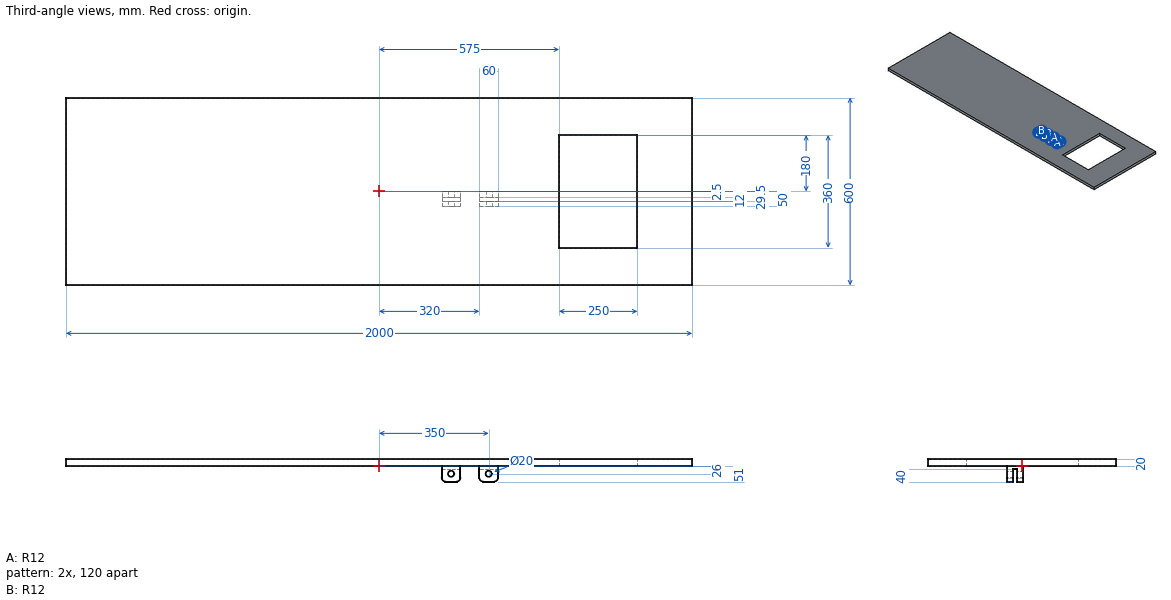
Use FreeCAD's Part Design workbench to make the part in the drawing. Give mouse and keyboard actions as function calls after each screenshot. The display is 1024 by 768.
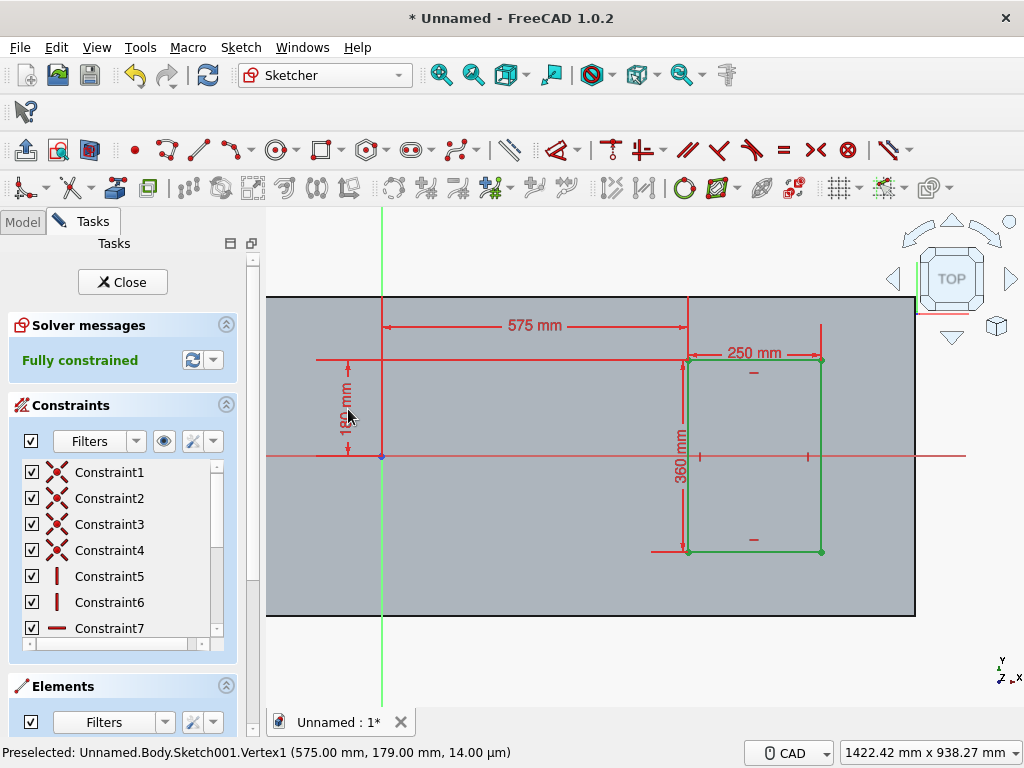
click(123, 282)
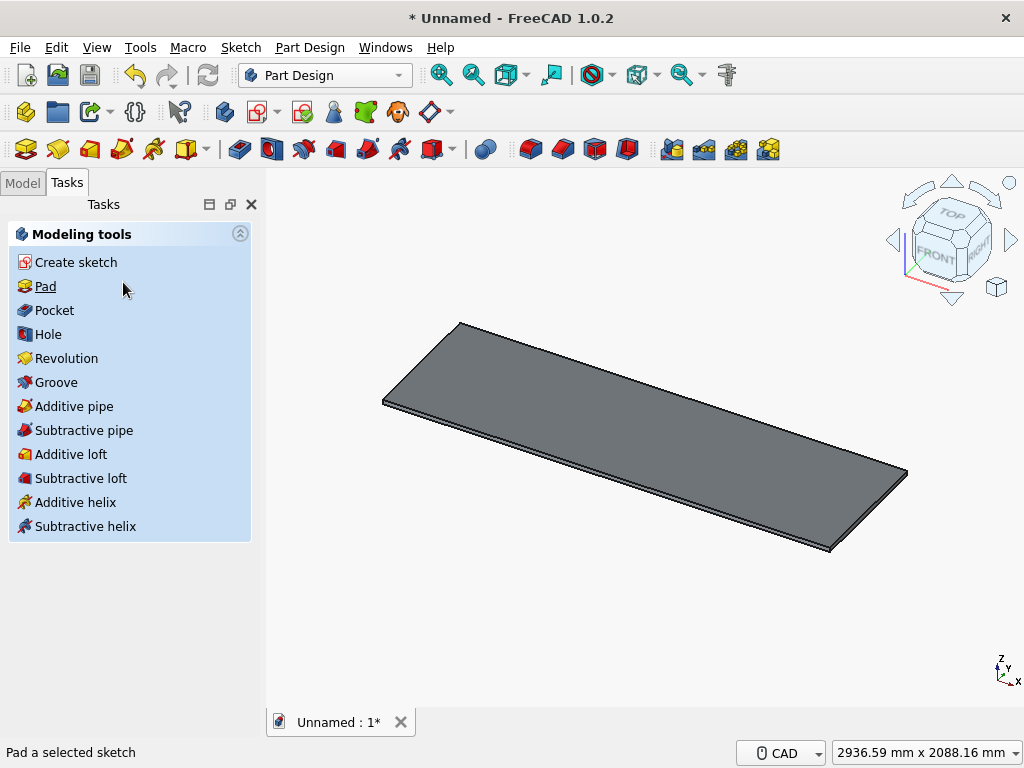
click(240, 150)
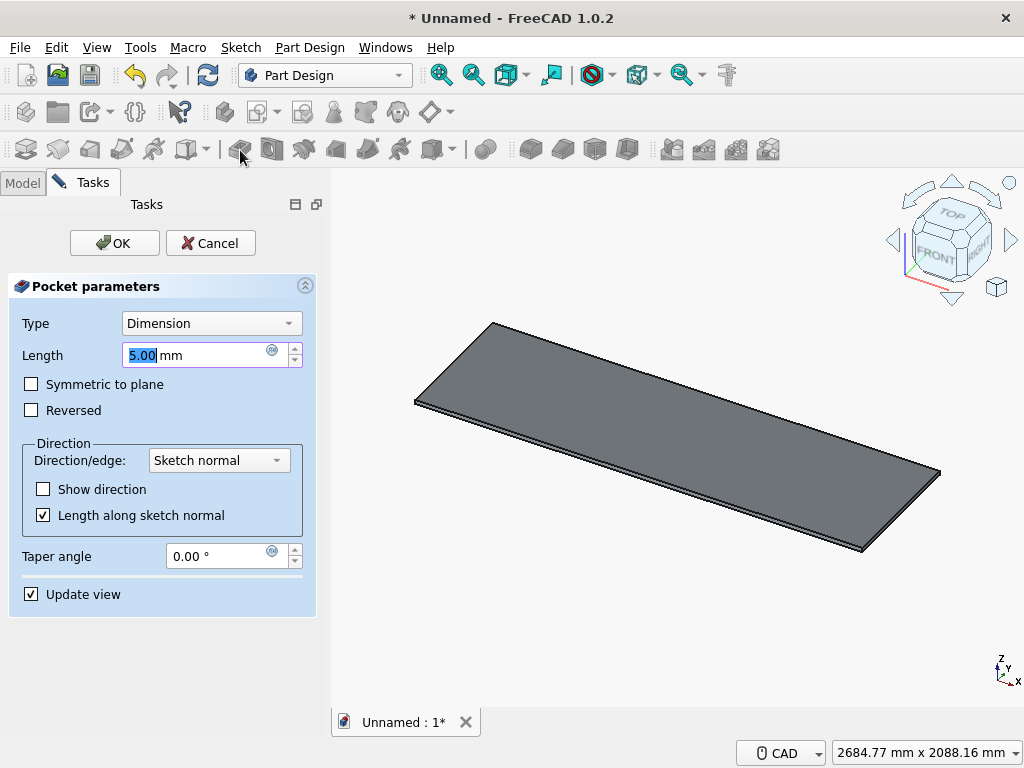
click(212, 324)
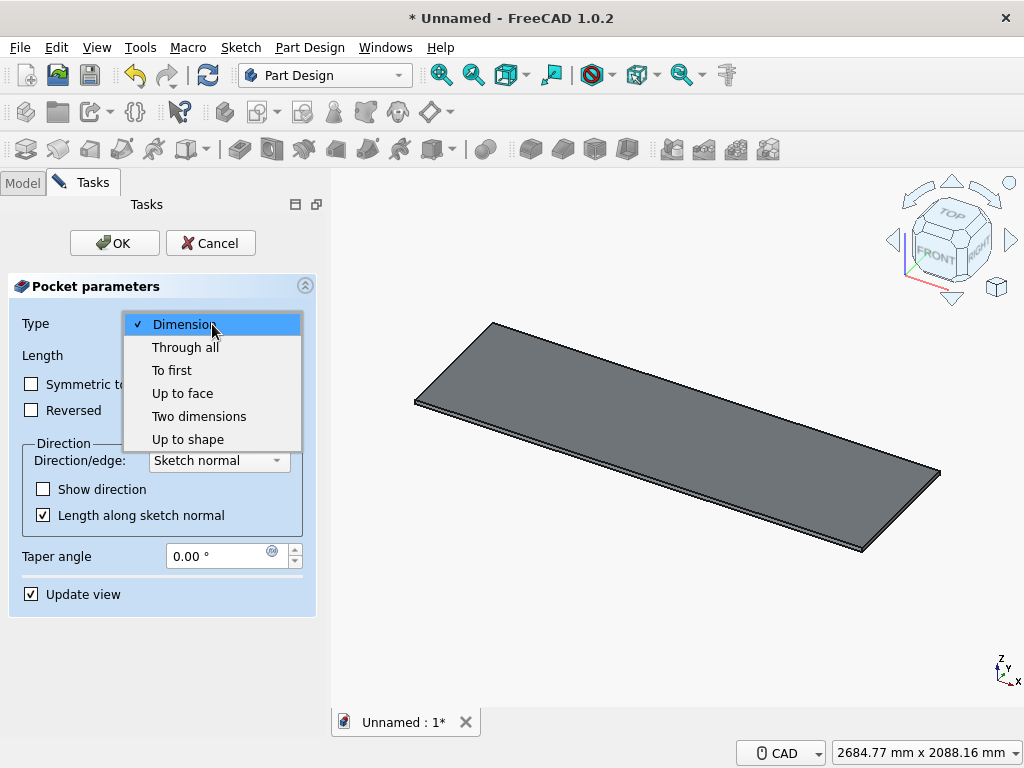
click(212, 348)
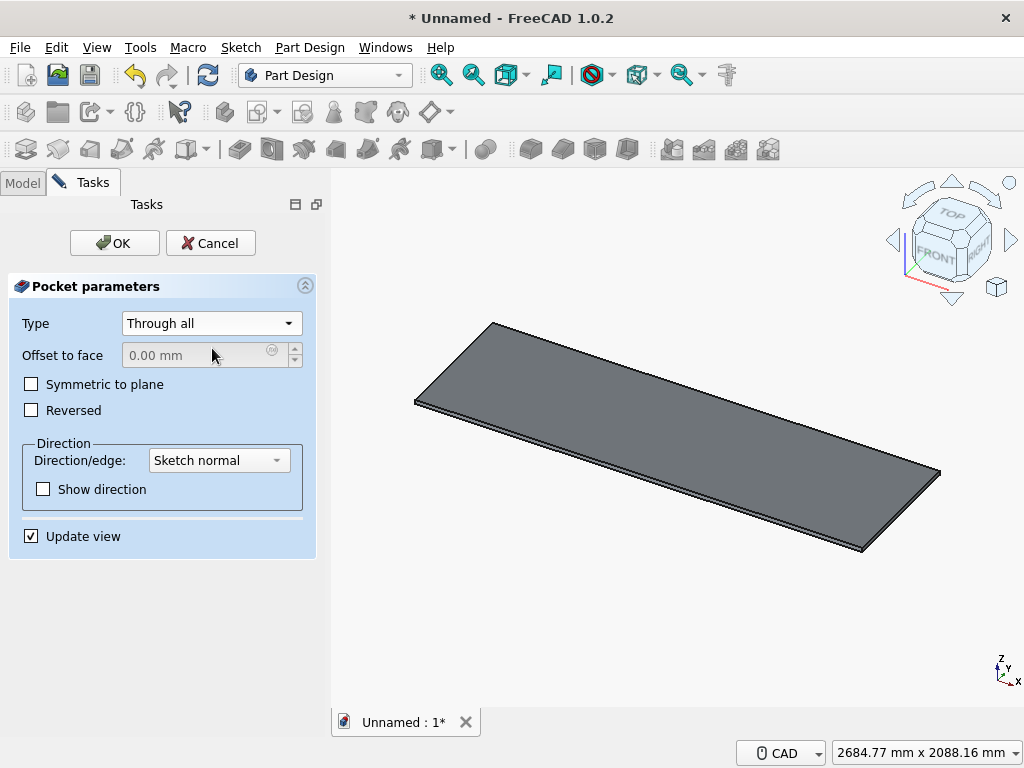
click(30, 410)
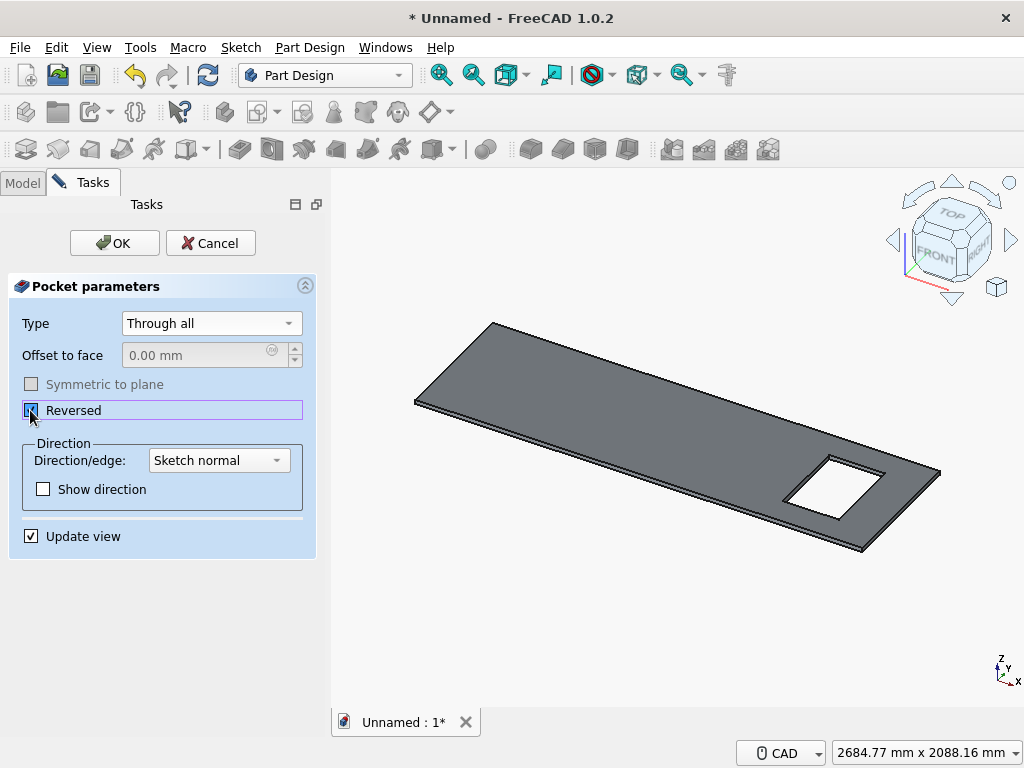
click(115, 243)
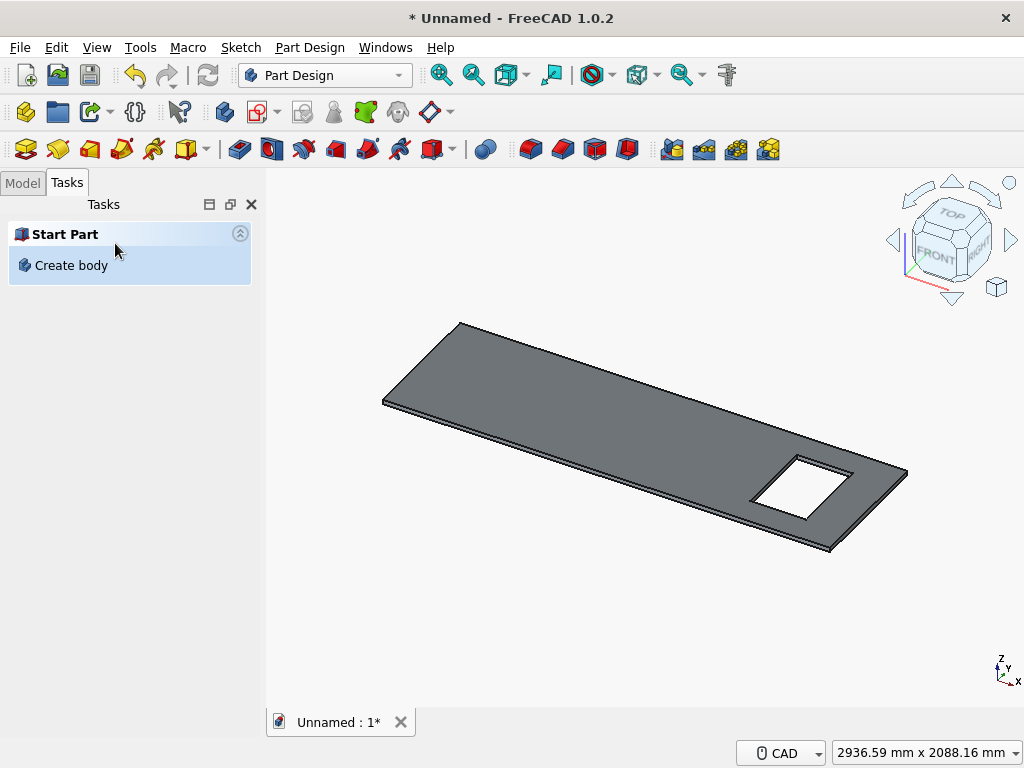
key(5)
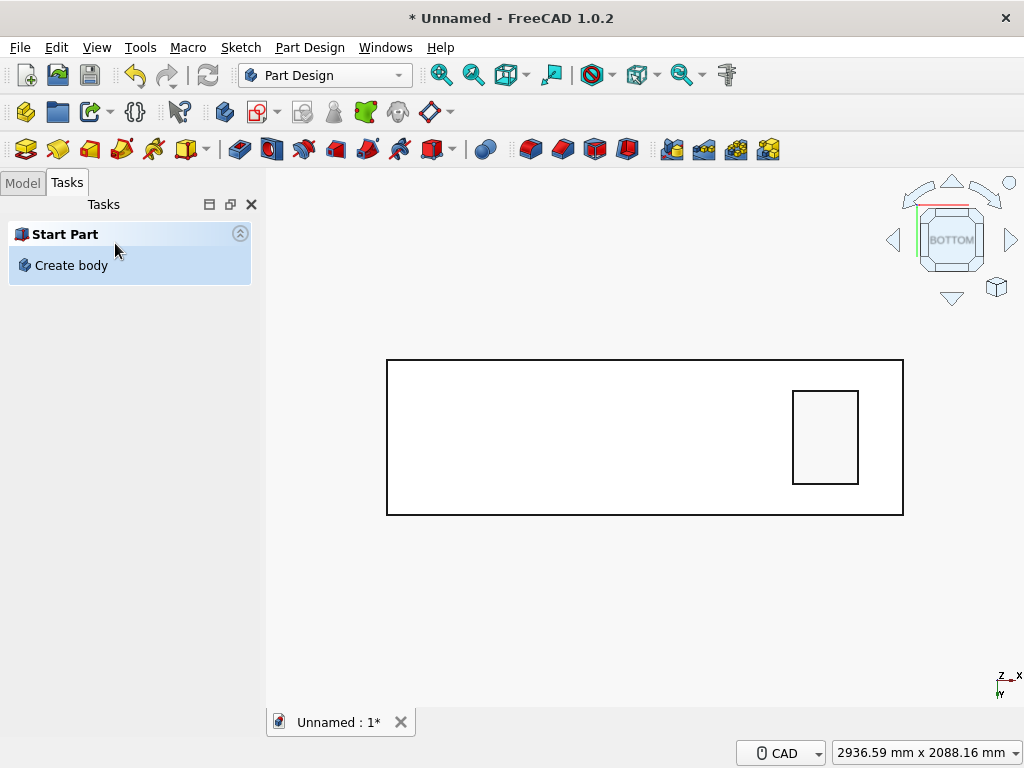
click(645, 436)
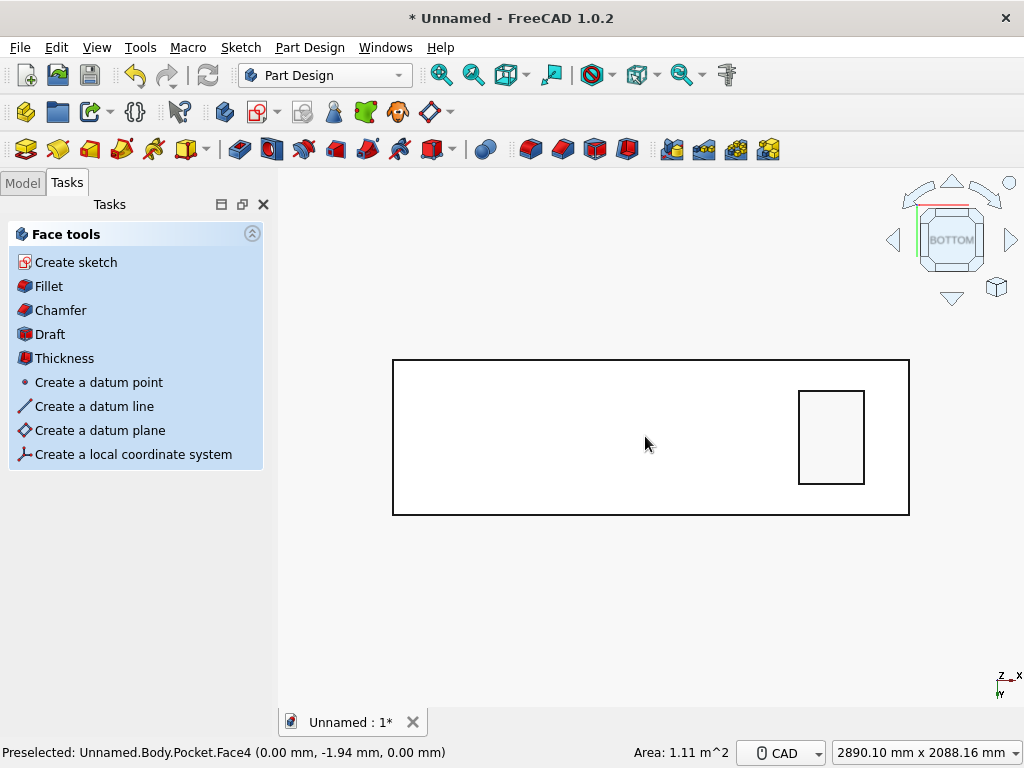
click(258, 112)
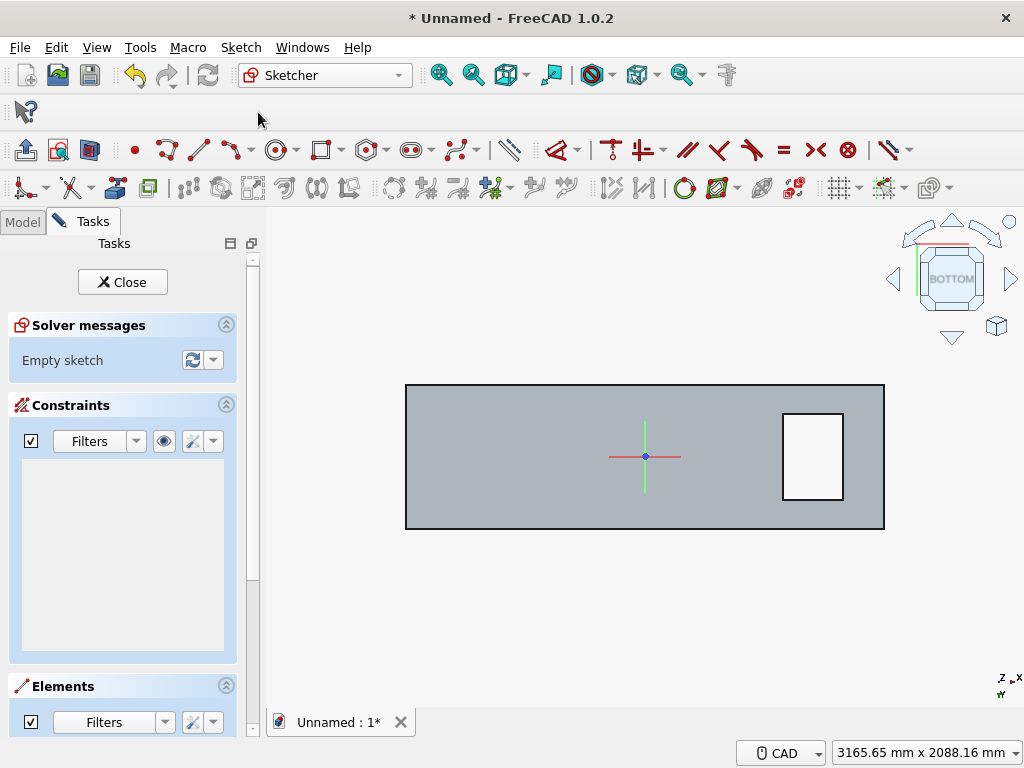
scroll(737, 451, up, 15)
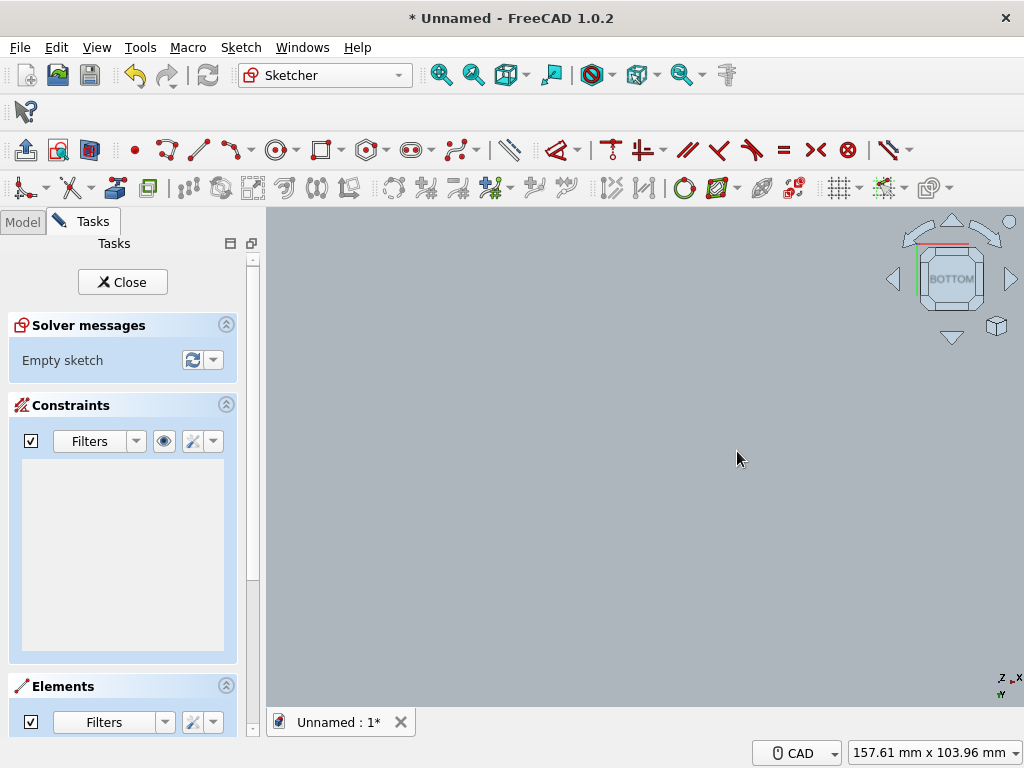
click(322, 150)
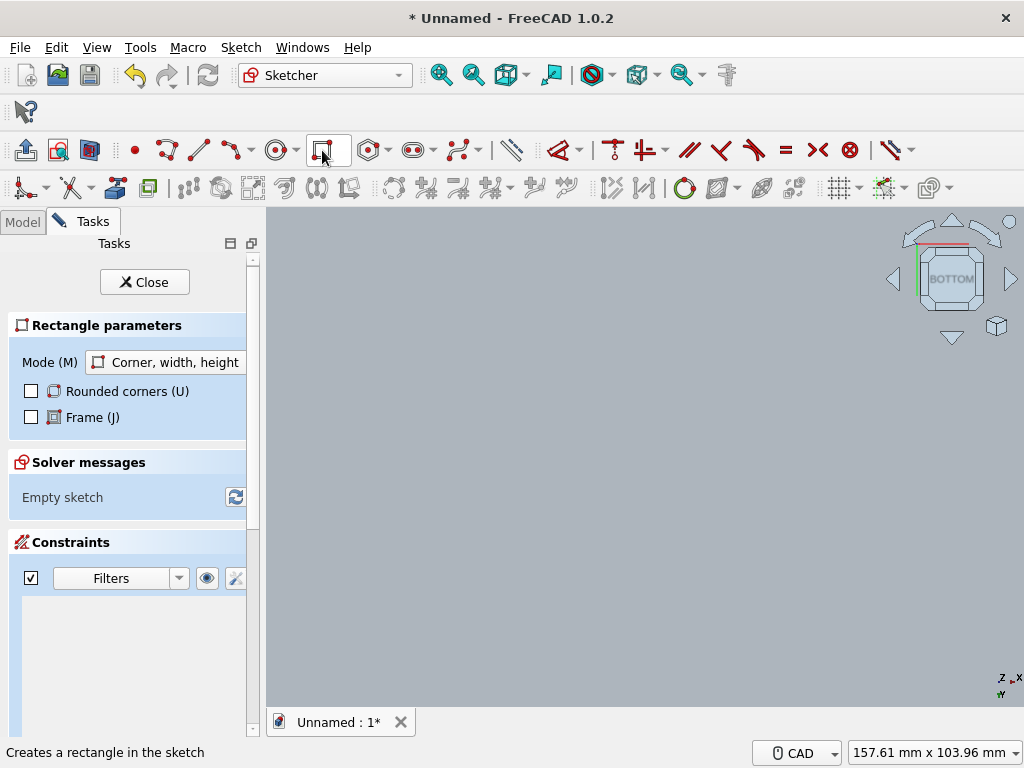
click(416, 334)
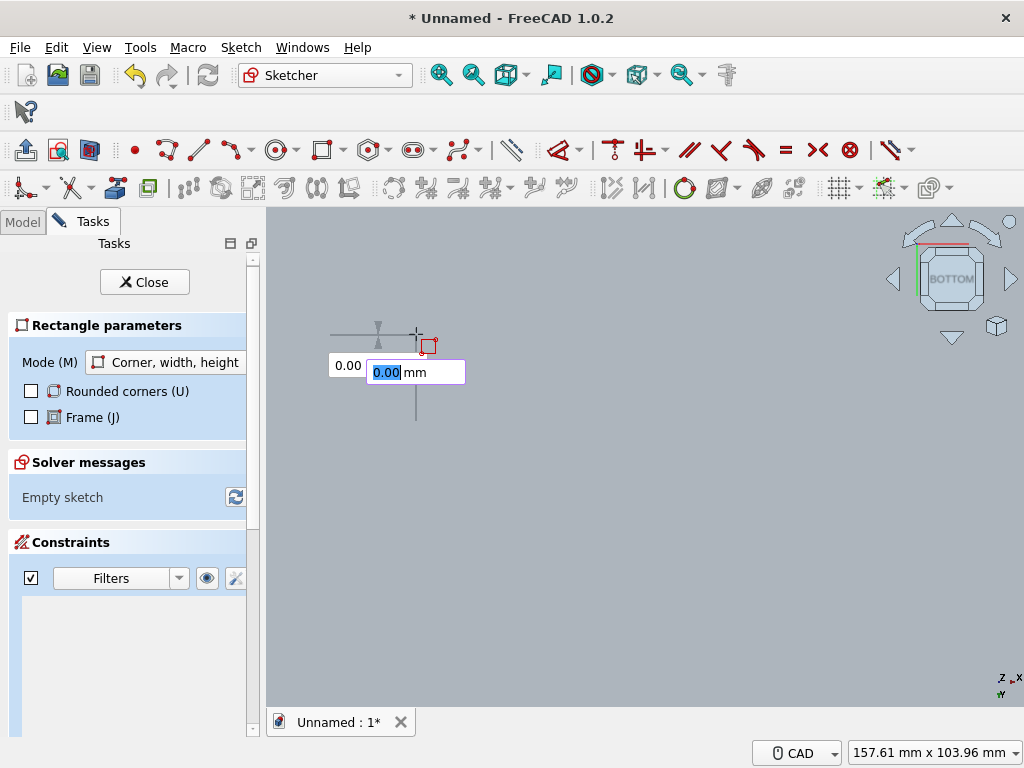
scroll(705, 574, up, 2)
move(704, 574)